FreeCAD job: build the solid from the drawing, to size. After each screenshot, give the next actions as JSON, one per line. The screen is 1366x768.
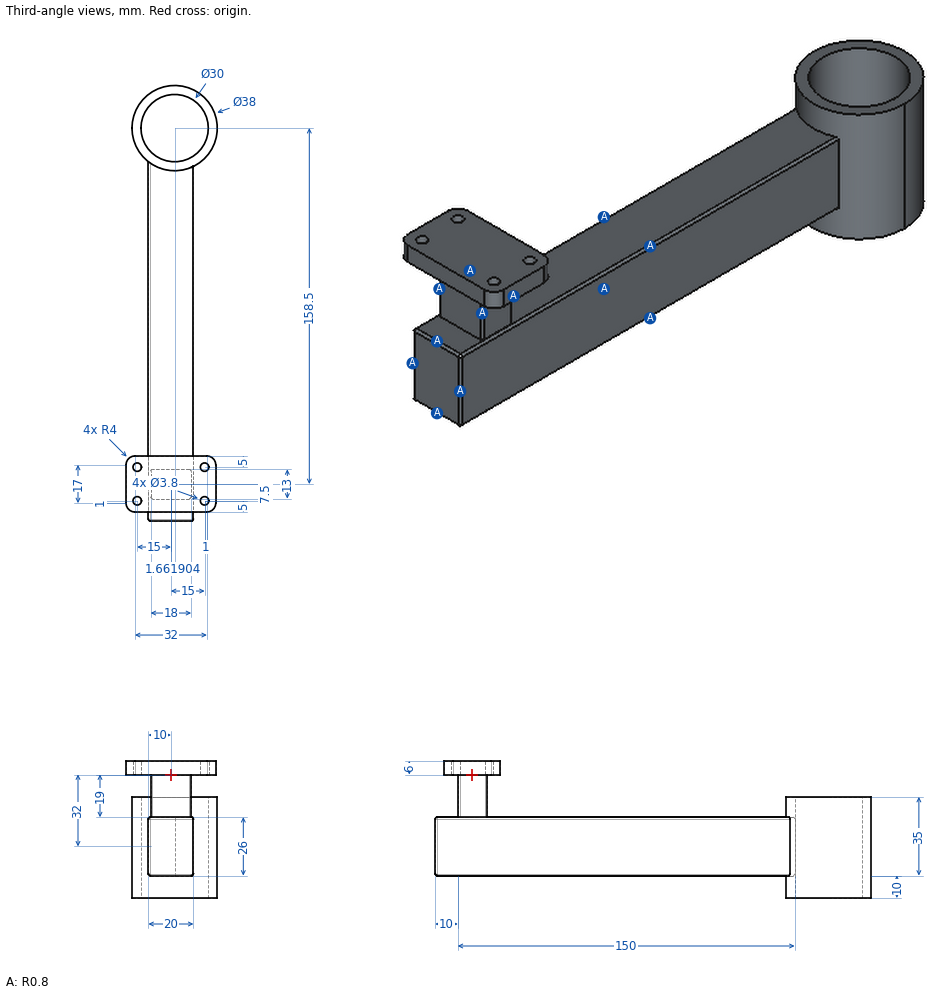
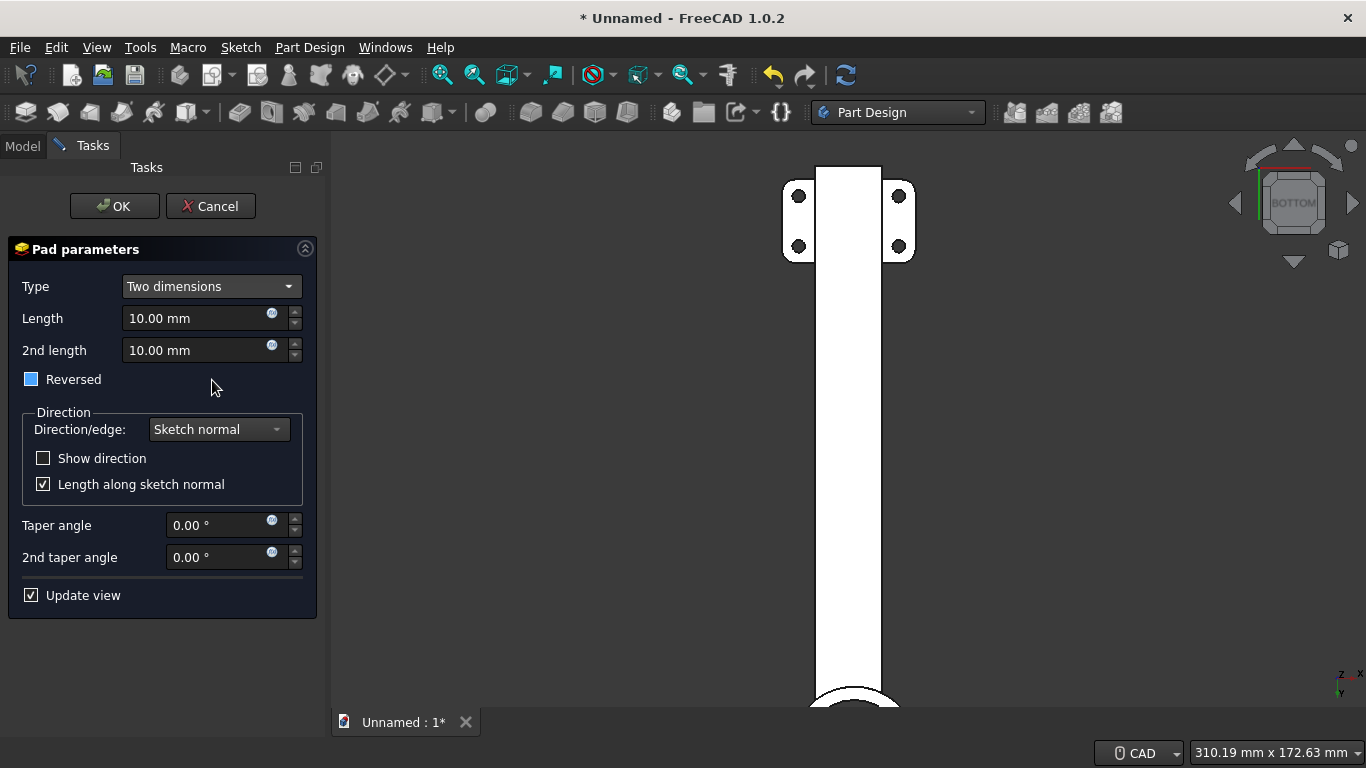
{"action": "triple_click", "coordinate": [204, 318]}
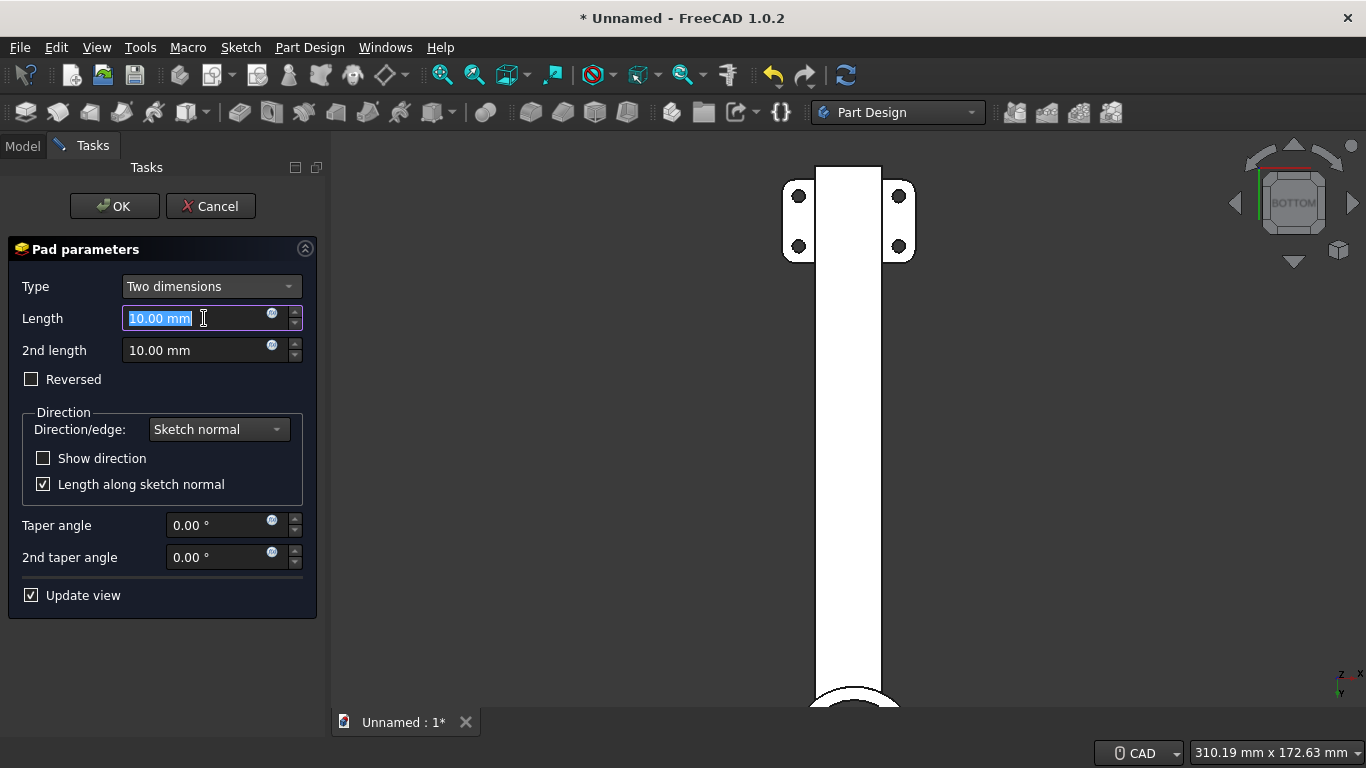
{"action": "type", "text": "10"}
{"action": "key", "text": "Tab"}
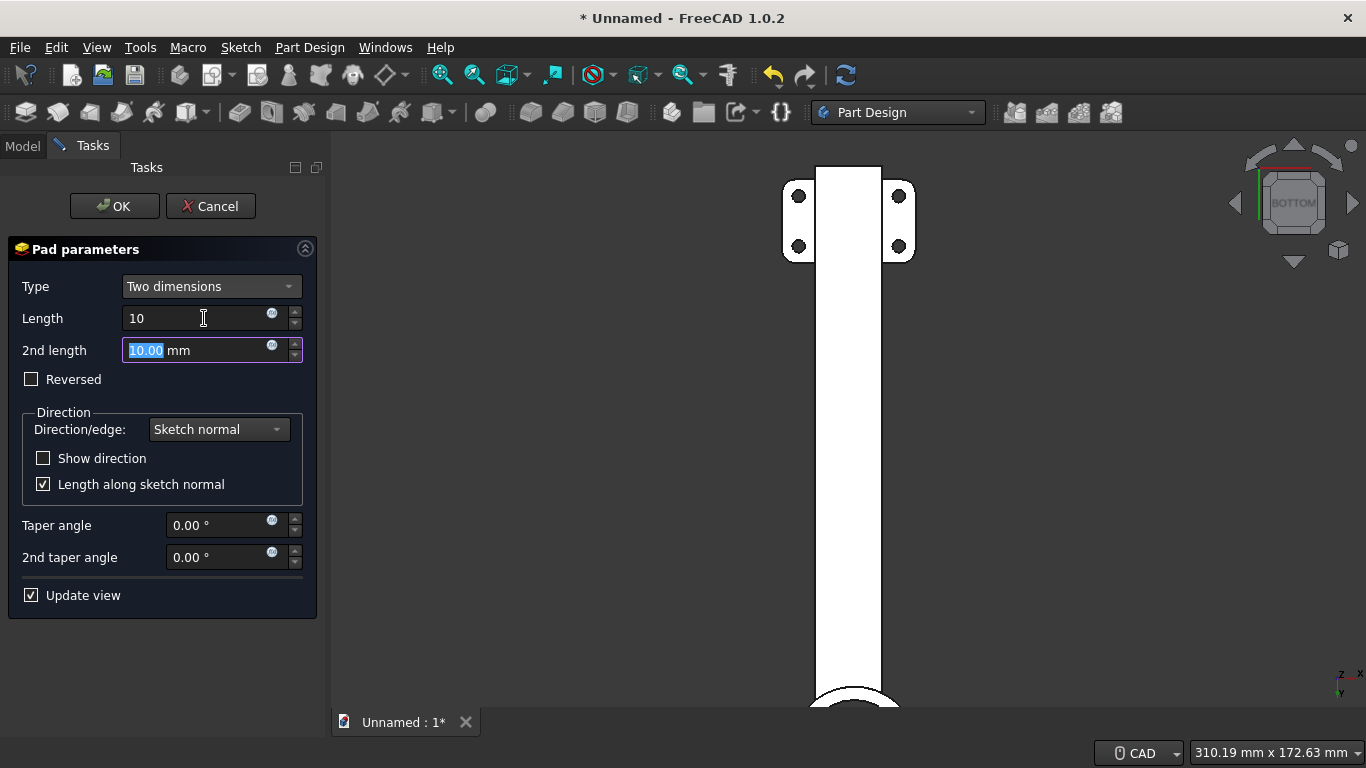
{"action": "type", "text": "35"}
{"action": "key", "text": "Tab"}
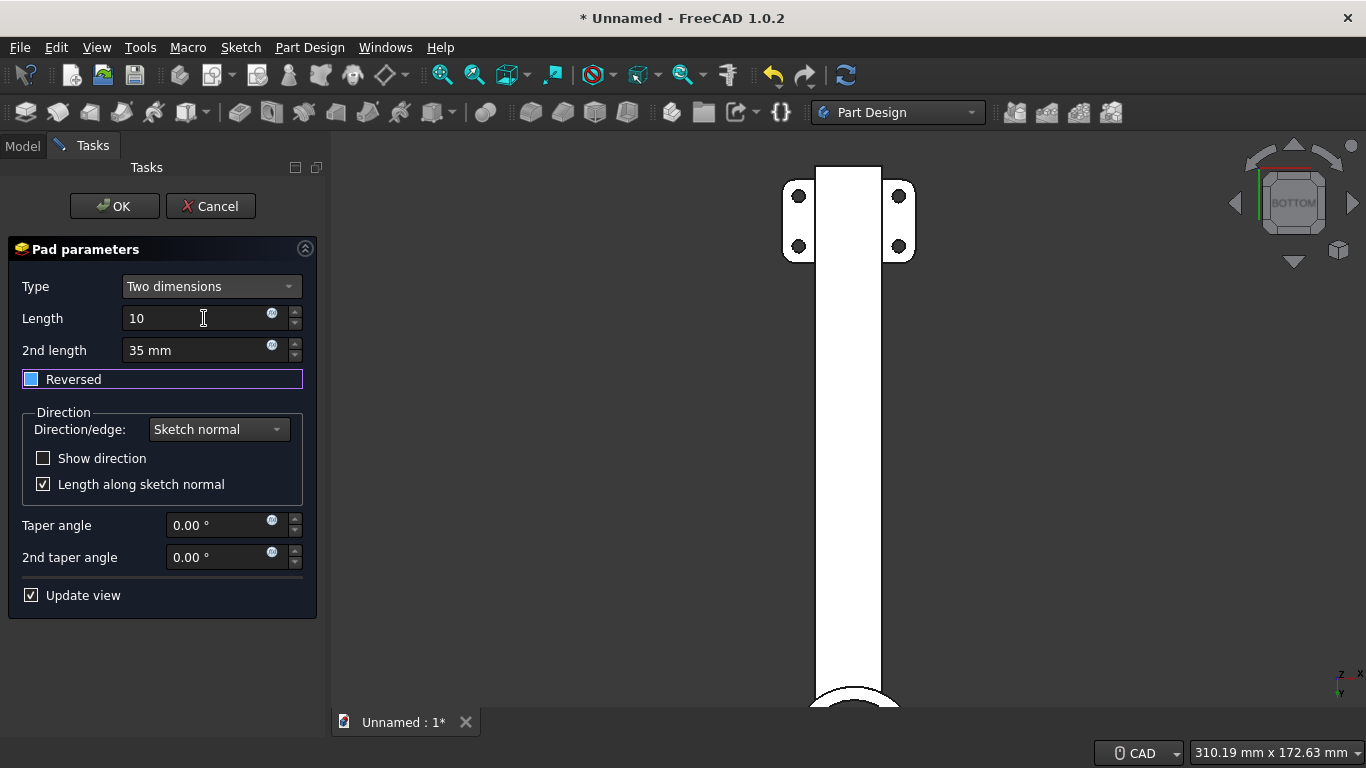
{"action": "left_click", "coordinate": [115, 206]}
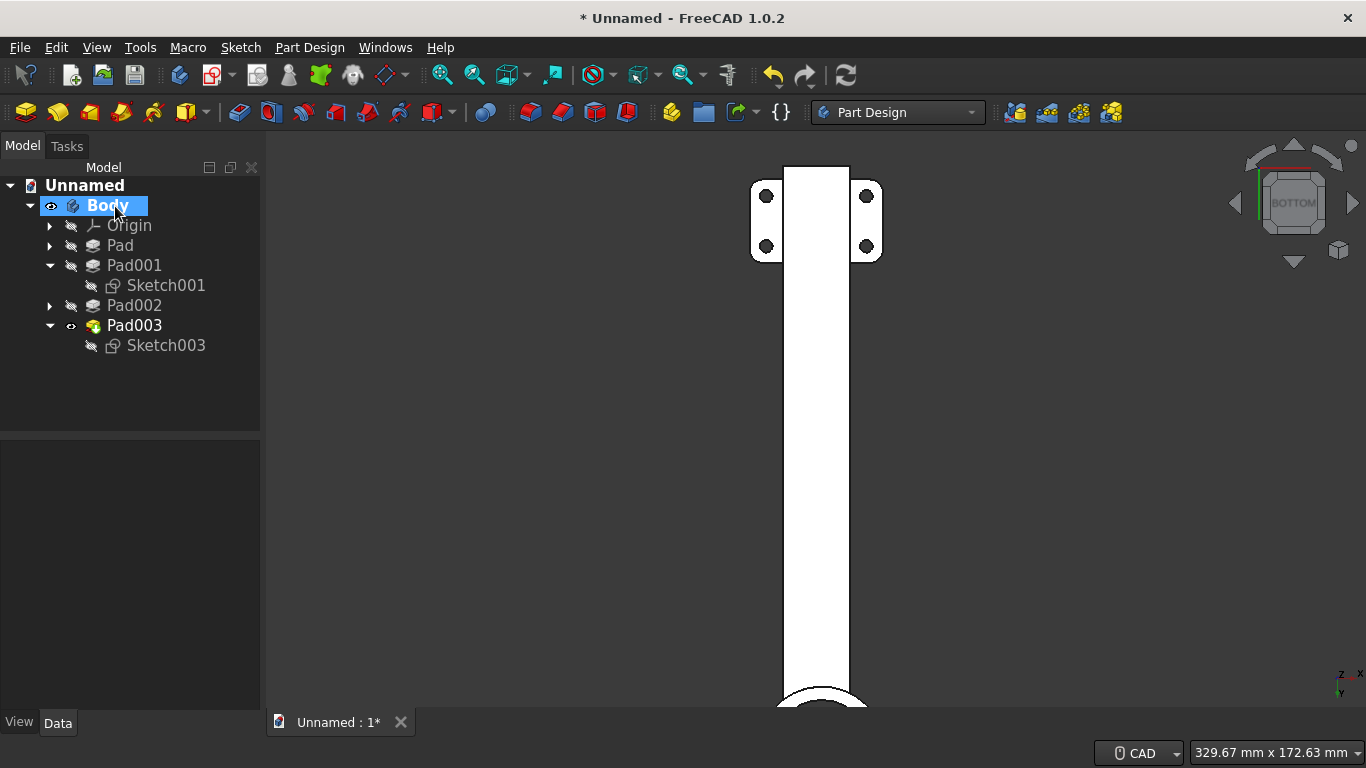
{"action": "key", "text": "v f"}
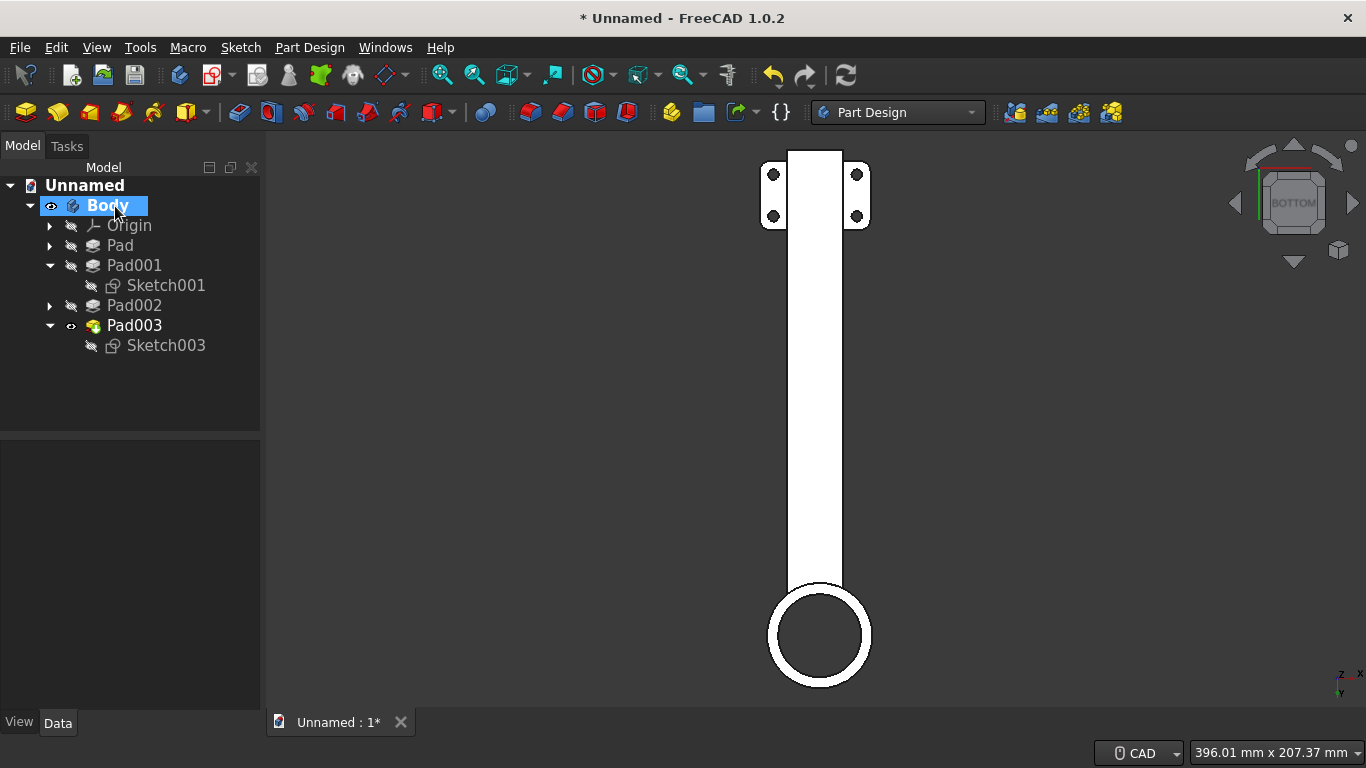
{"action": "left_click", "coordinate": [787, 371]}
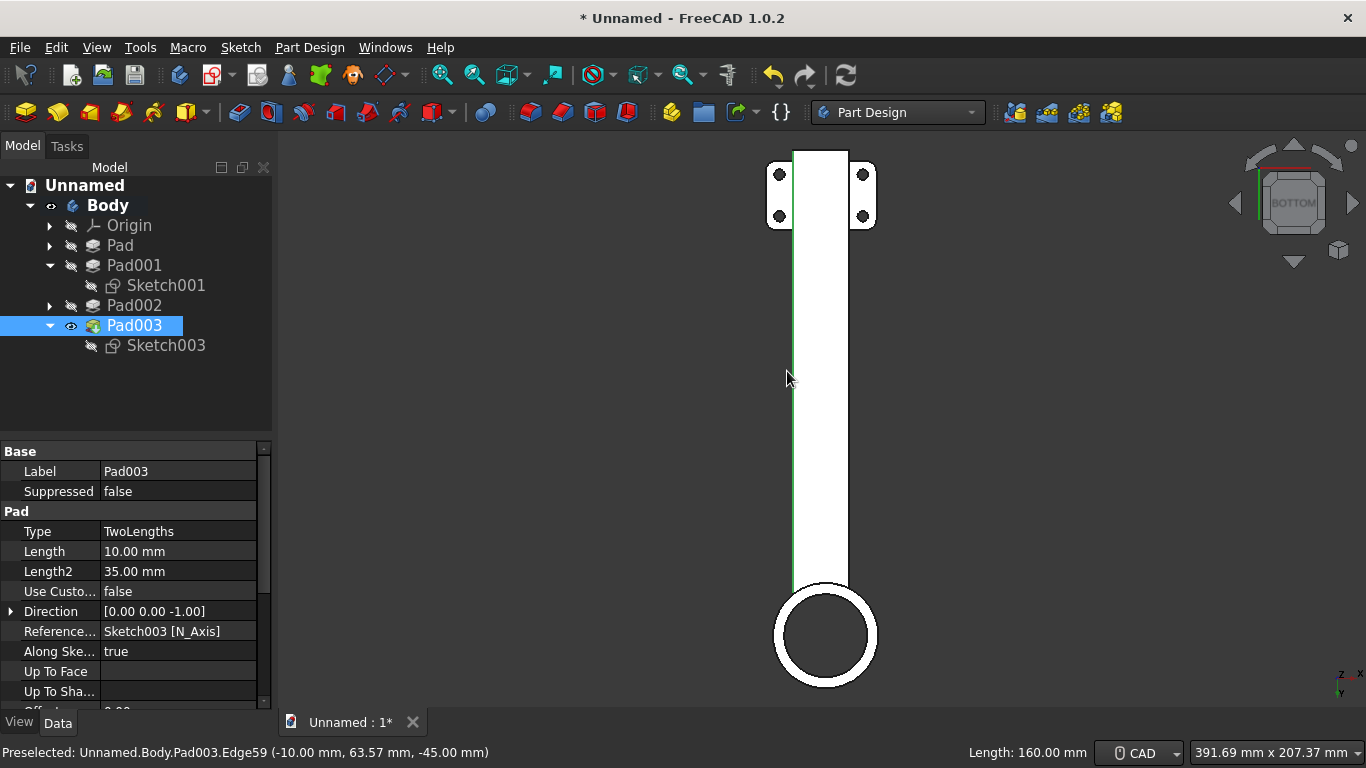
{"action": "left_click", "coordinate": [849, 368], "text": "ctrl"}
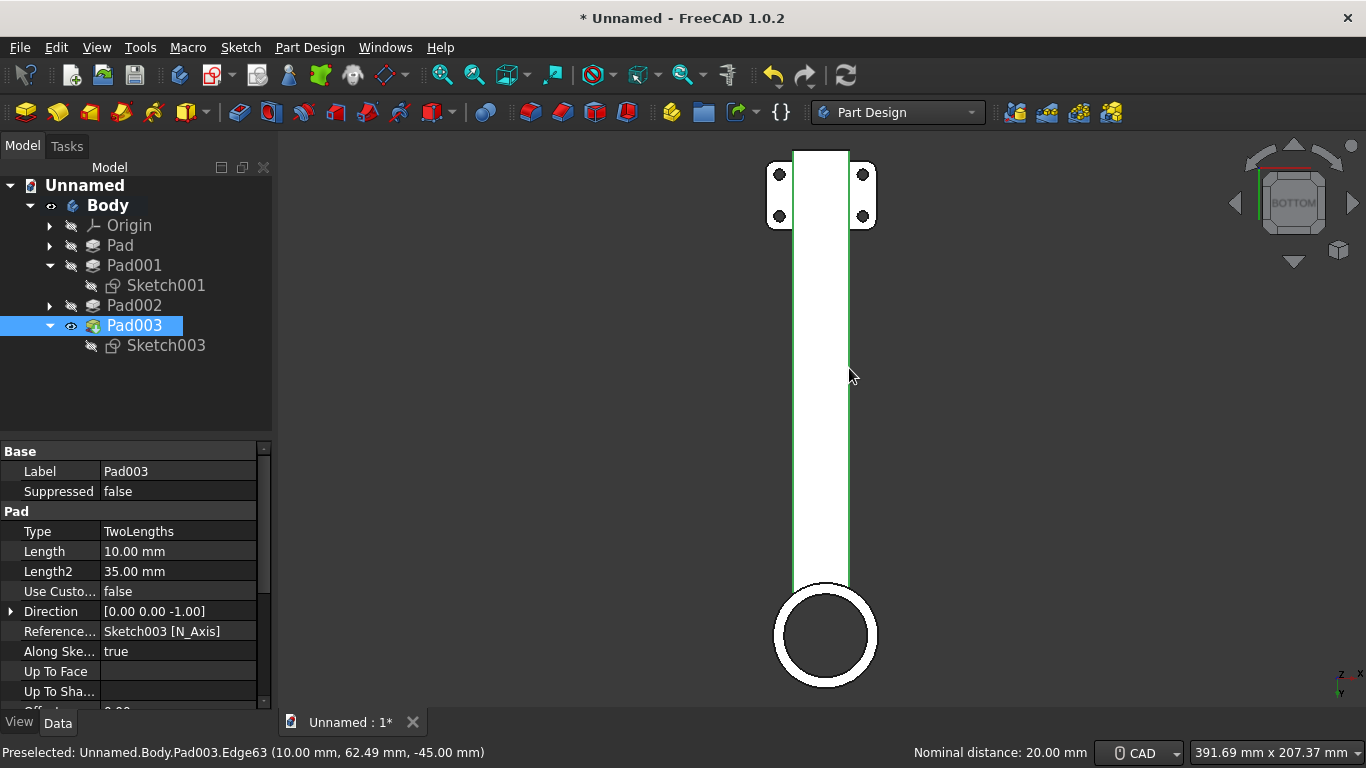
{"action": "key", "text": "0"}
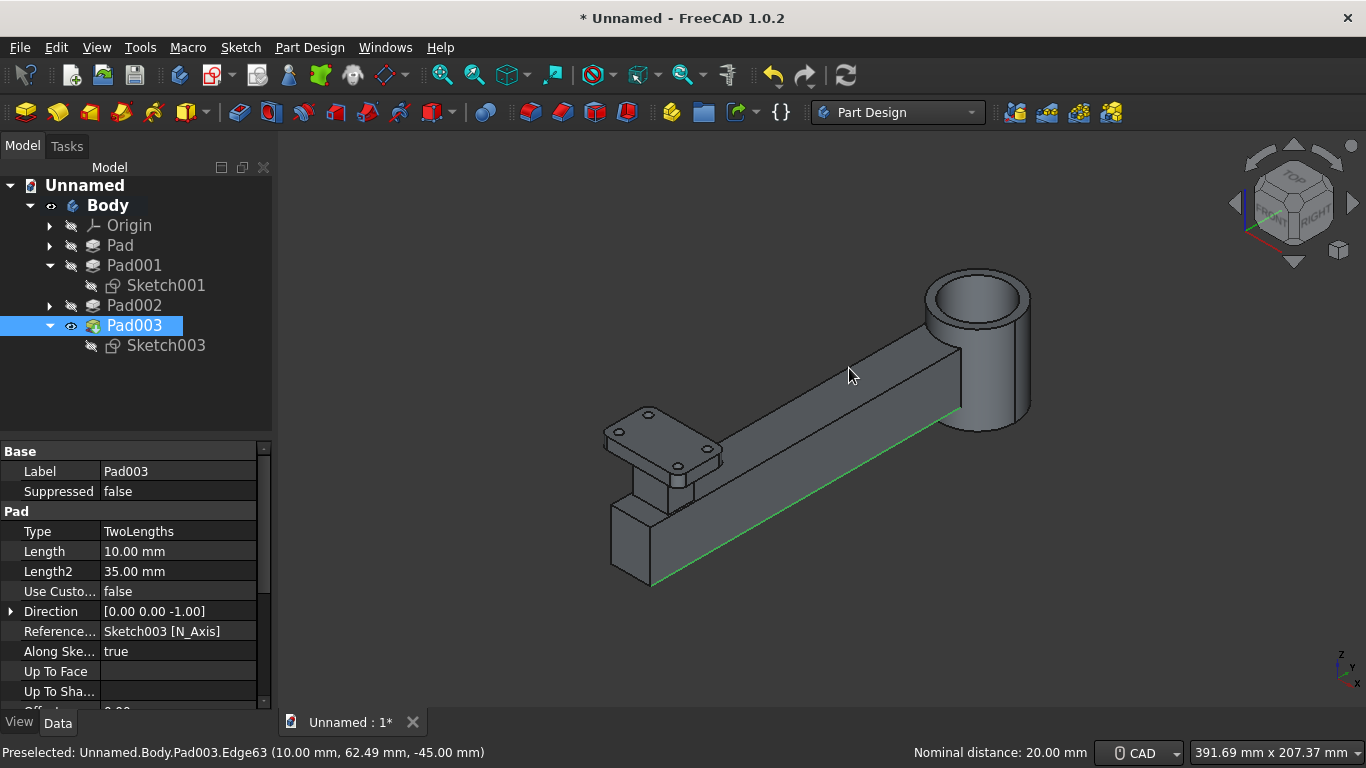
{"action": "left_click", "coordinate": [631, 545], "text": "ctrl"}